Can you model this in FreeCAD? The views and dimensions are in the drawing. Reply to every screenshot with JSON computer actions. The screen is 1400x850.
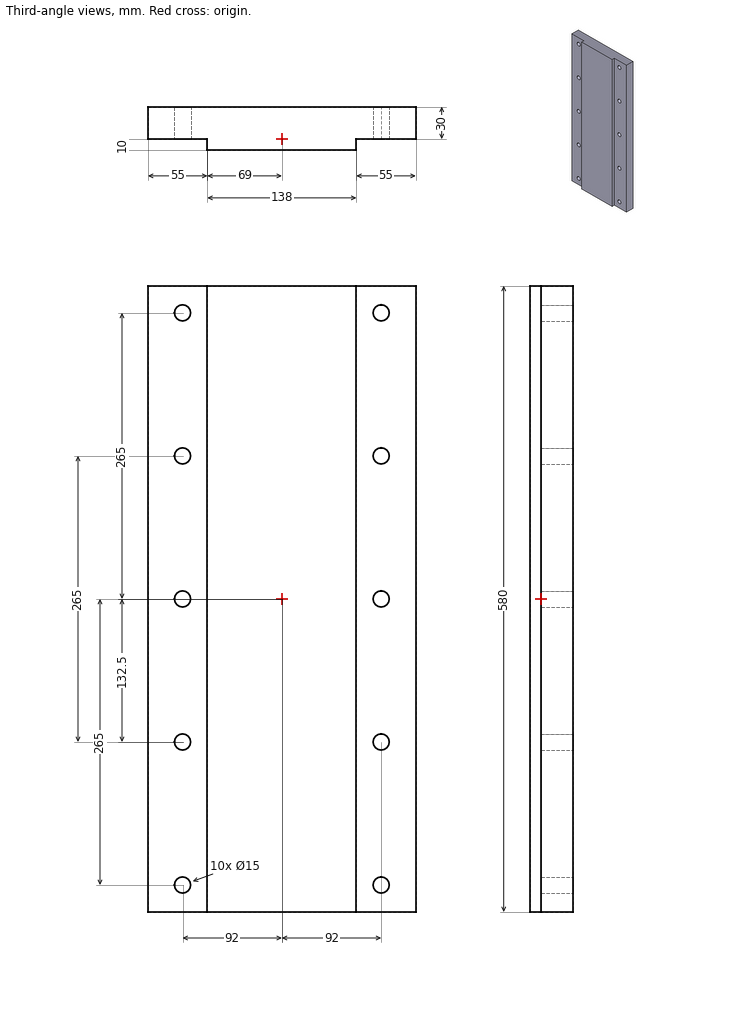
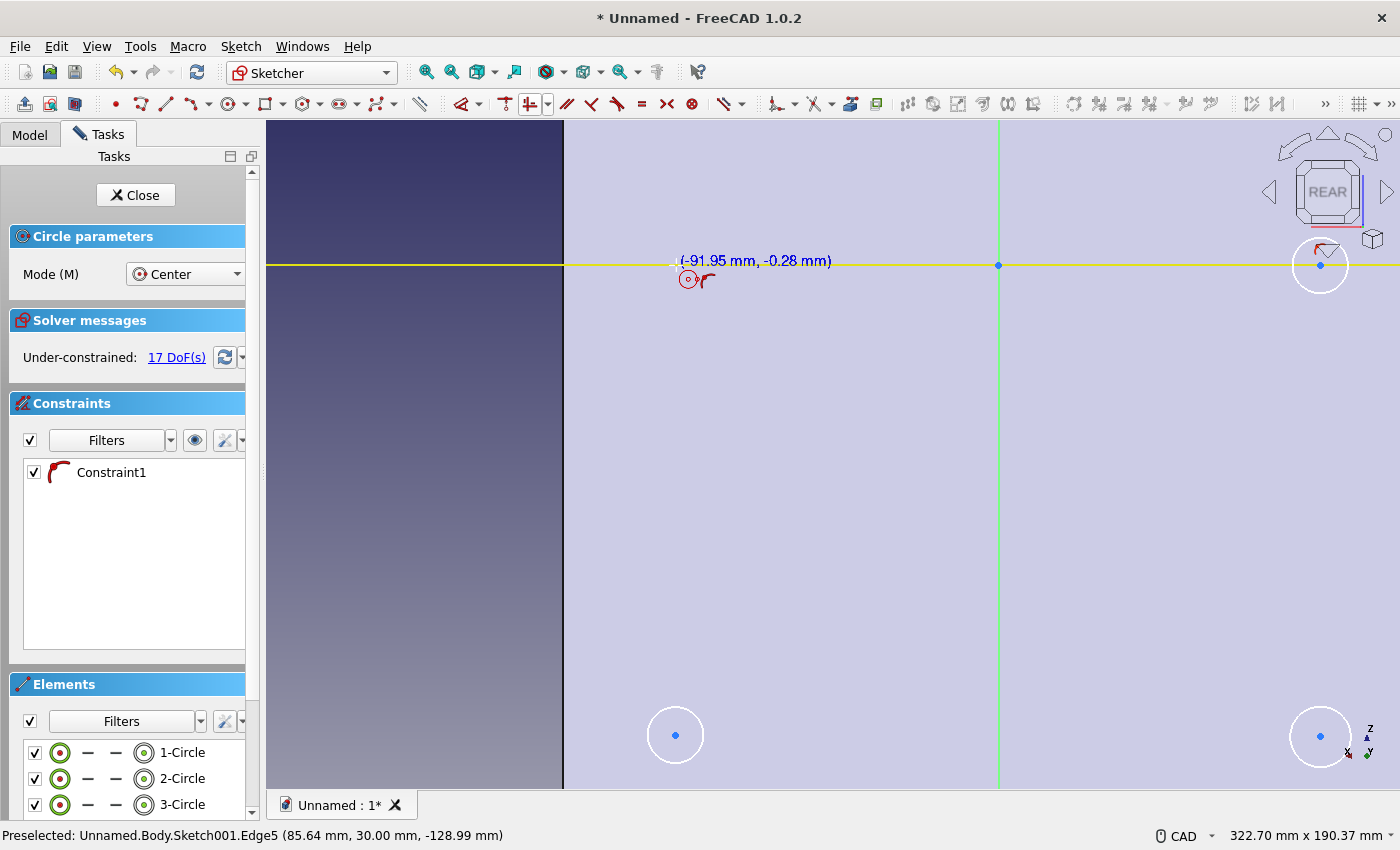
{"action": "scroll", "coordinate": [688, 516], "scroll_direction": "down", "scroll_amount": 7}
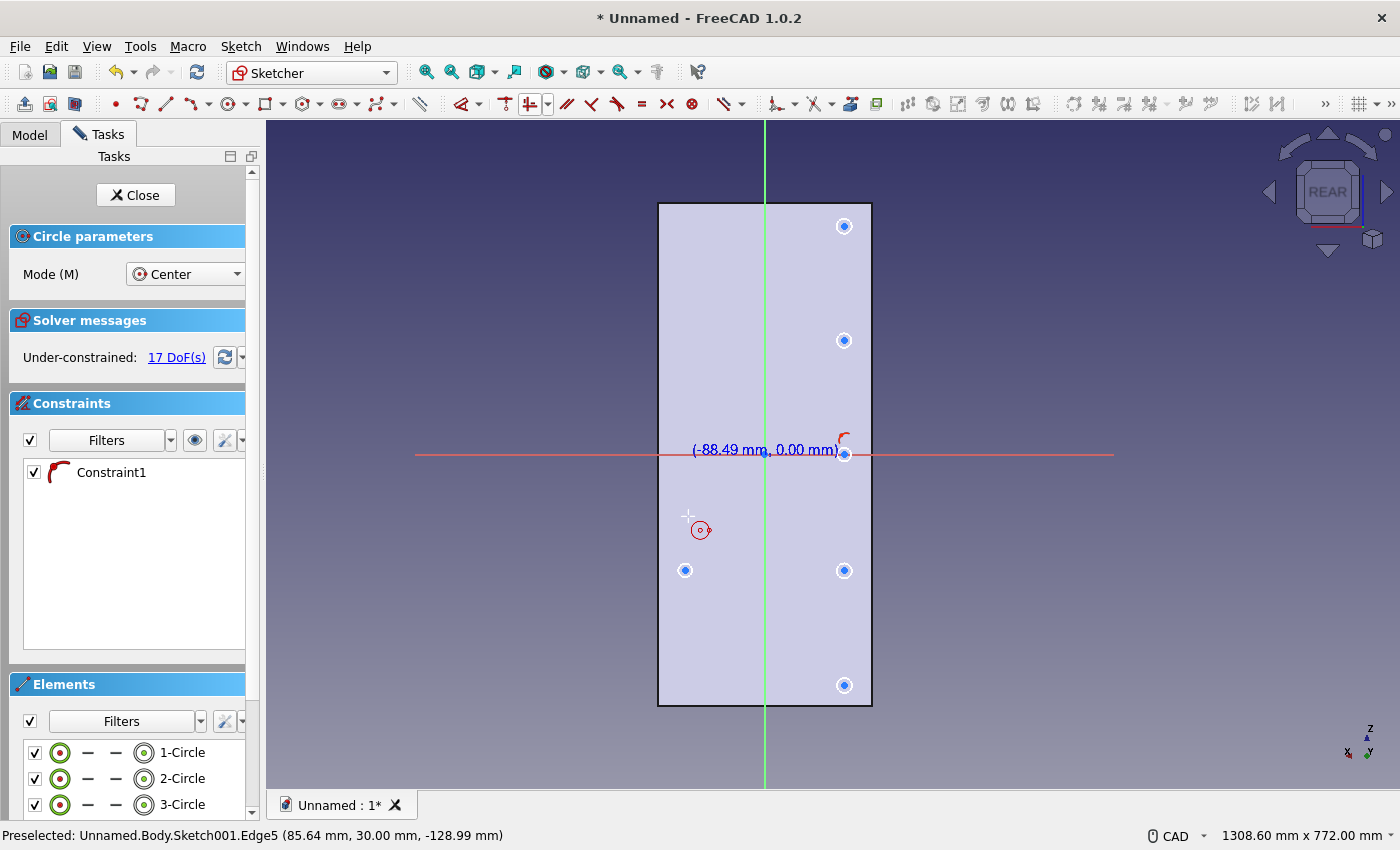
{"action": "left_click", "coordinate": [685, 455]}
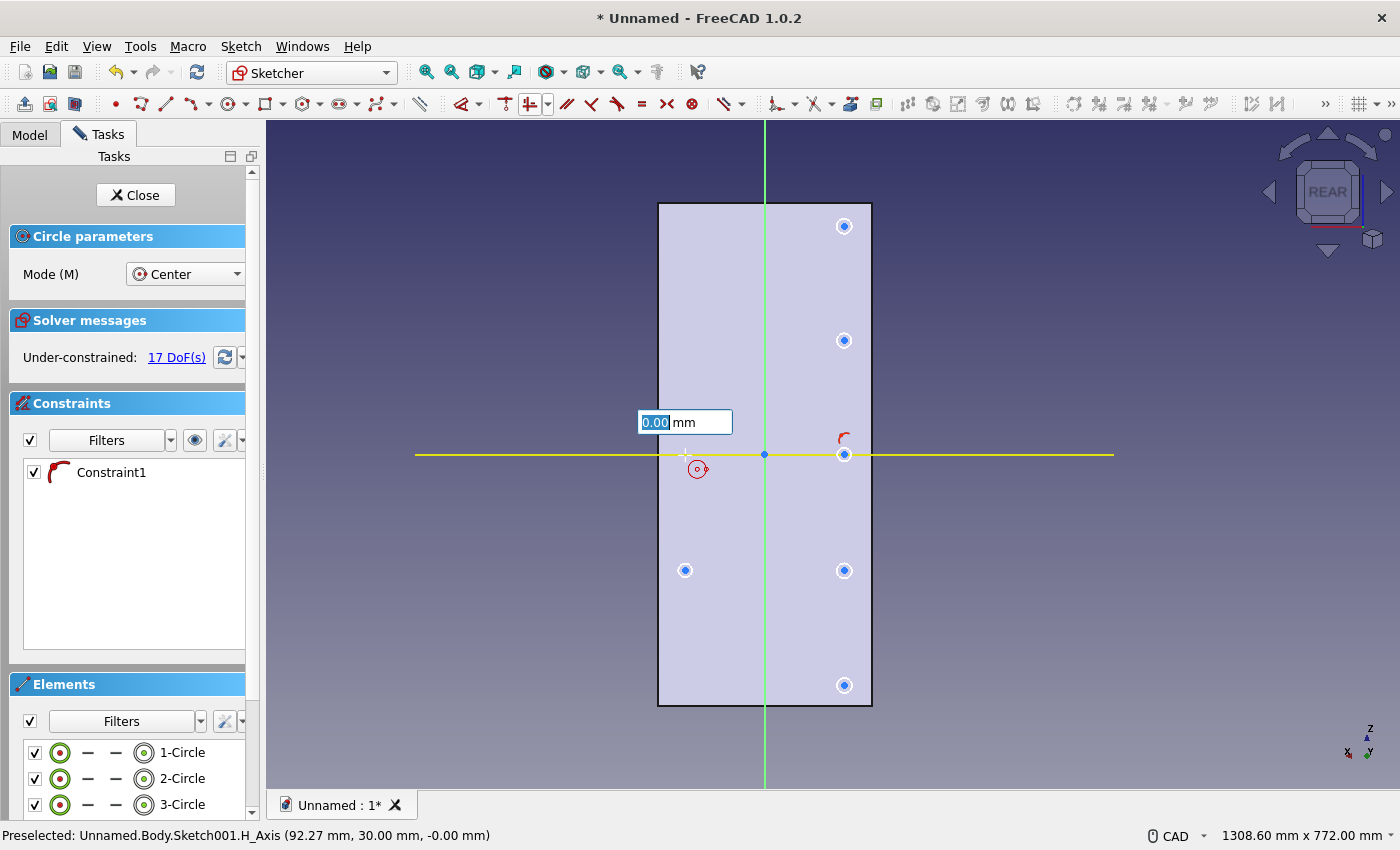
{"action": "scroll", "coordinate": [683, 461], "scroll_direction": "up", "scroll_amount": 5}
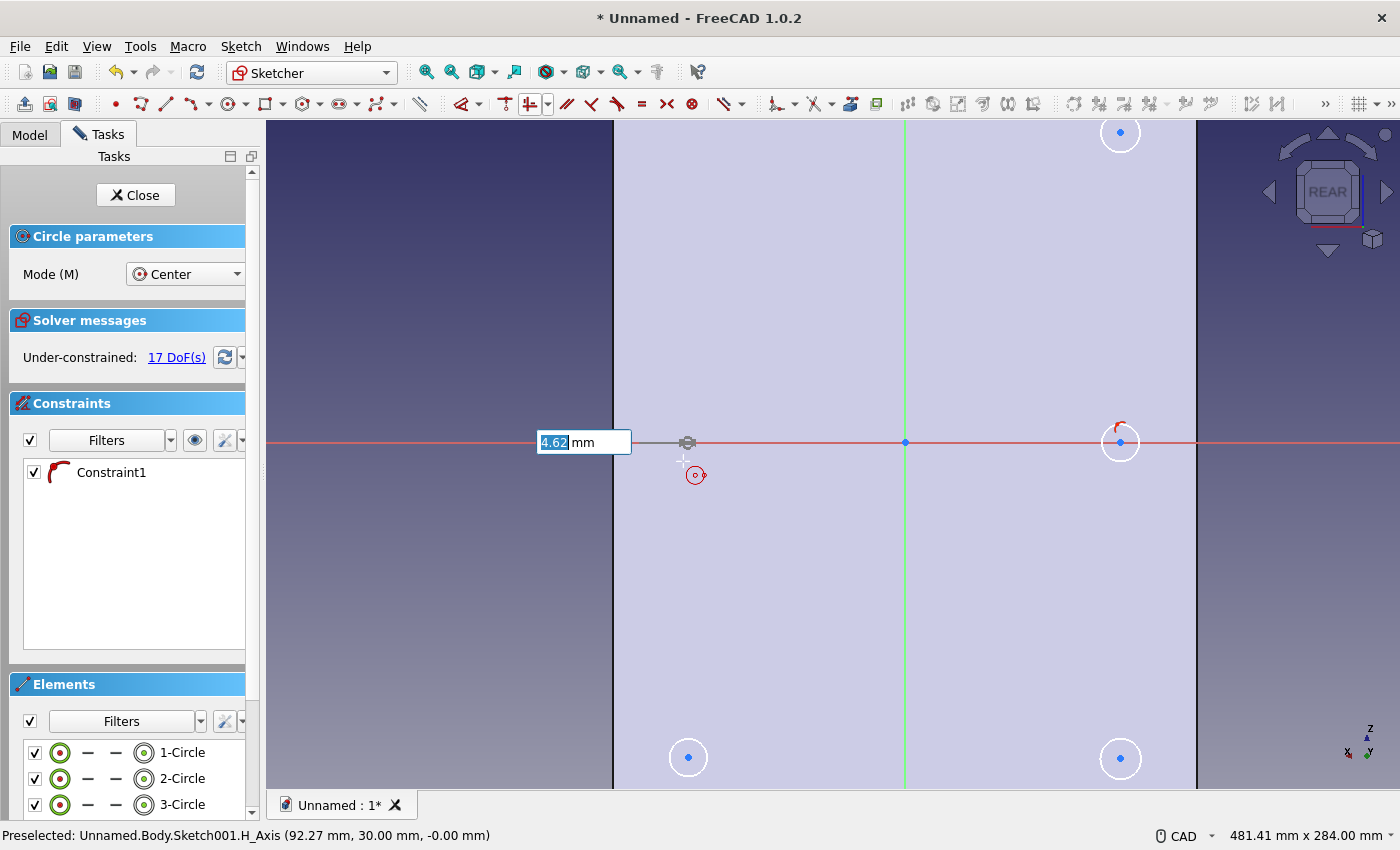
{"action": "left_click", "coordinate": [682, 459]}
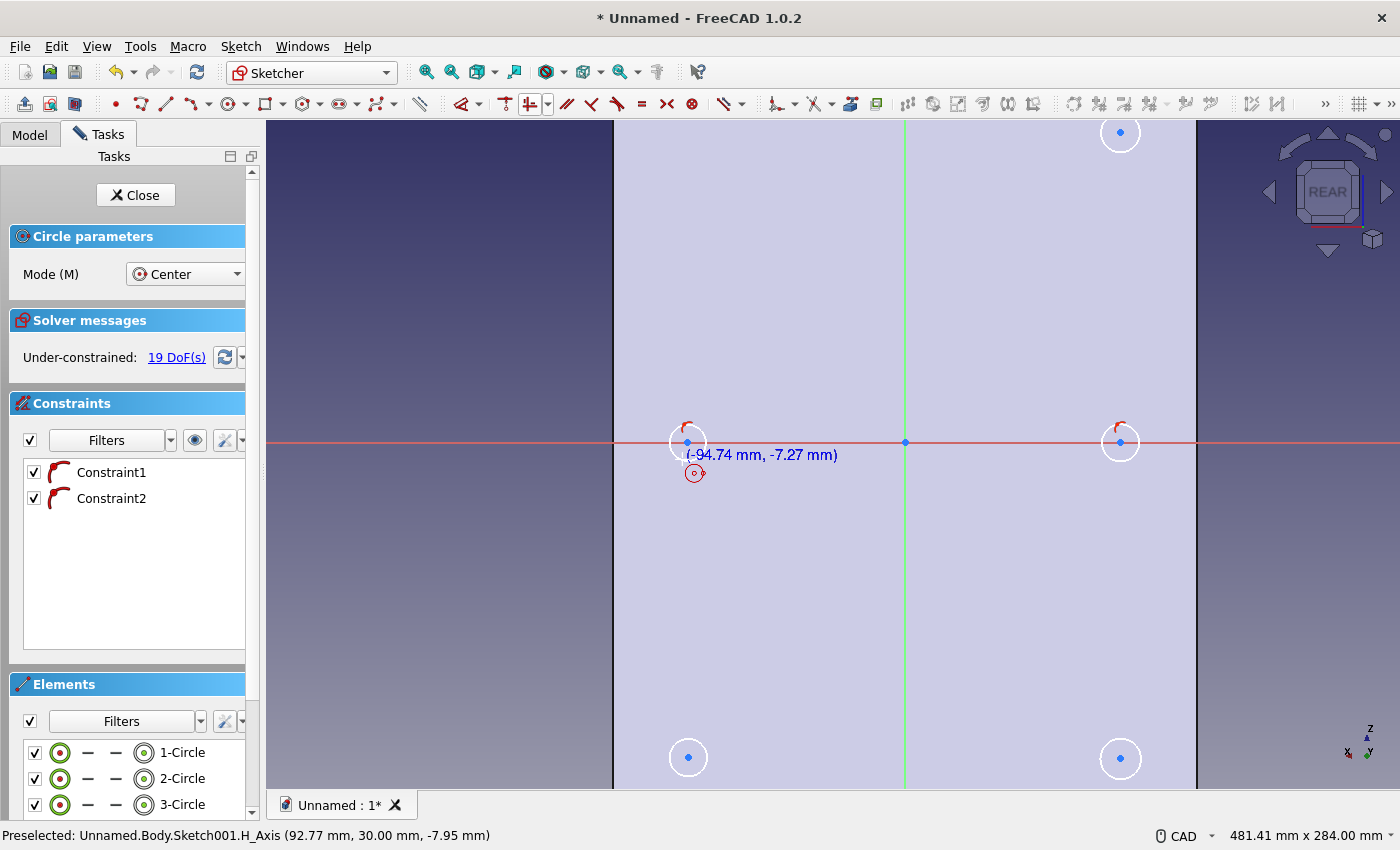
{"action": "scroll", "coordinate": [683, 461], "scroll_direction": "down", "scroll_amount": 5}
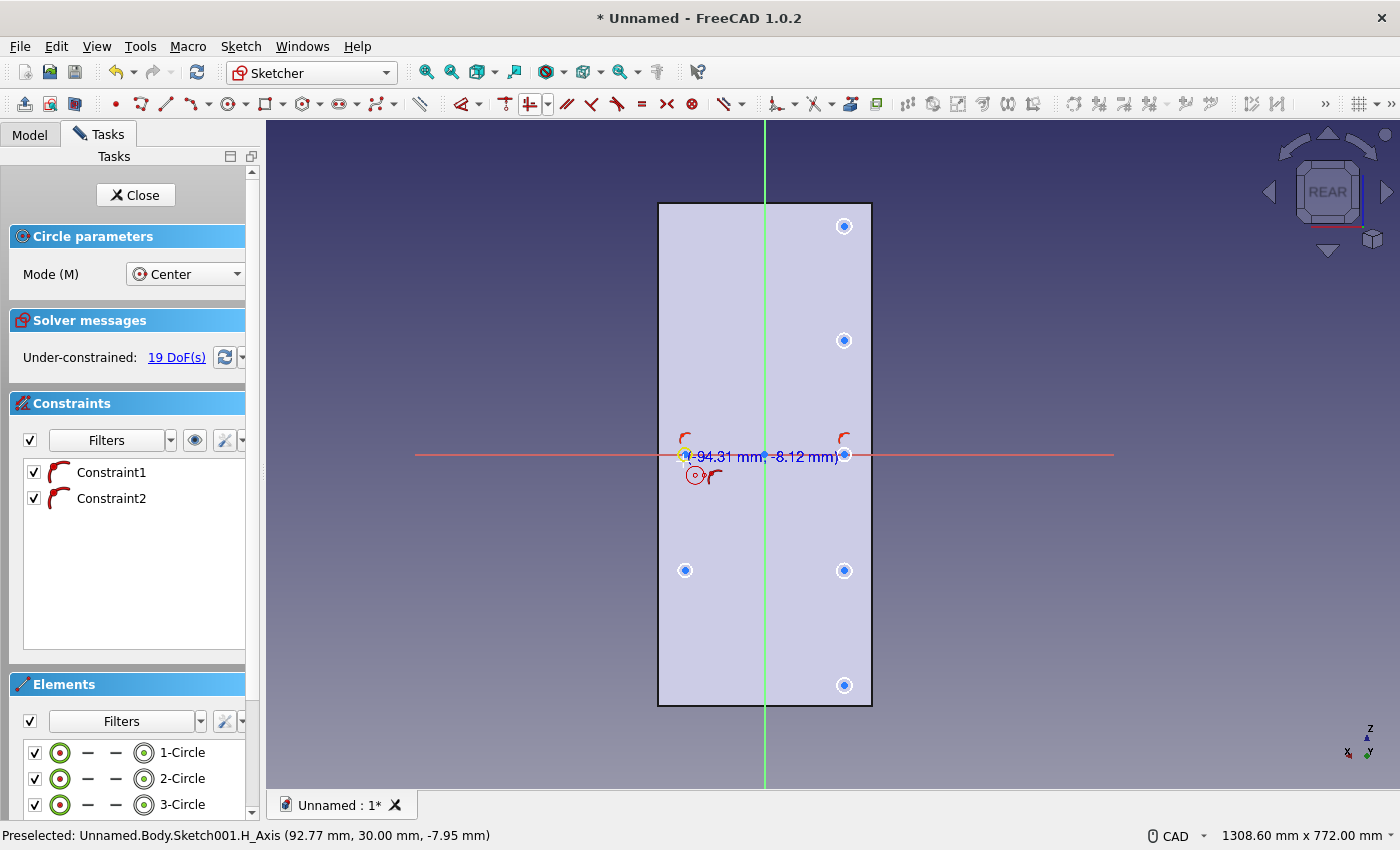
{"action": "scroll", "coordinate": [685, 340], "scroll_direction": "up", "scroll_amount": 7}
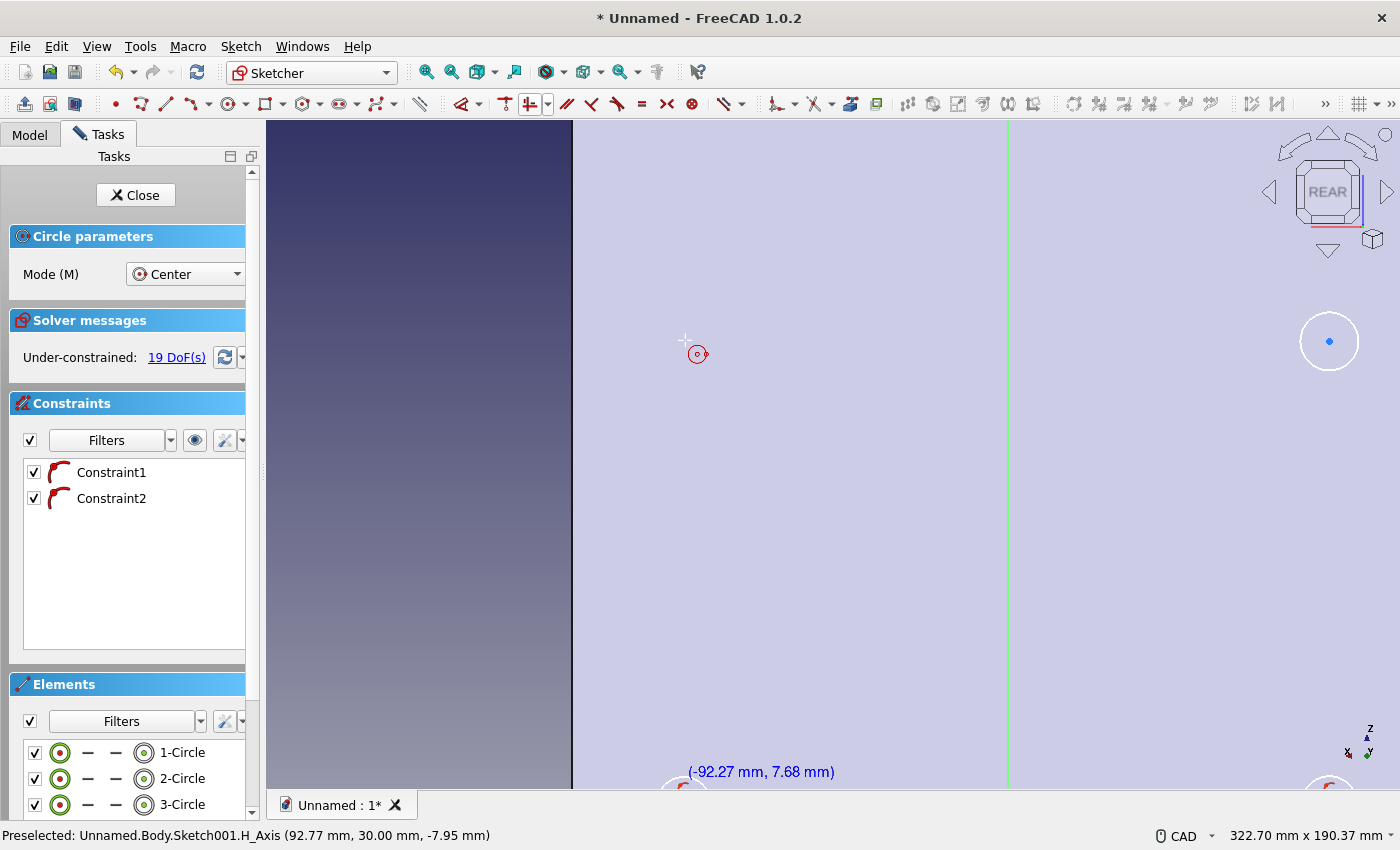
{"action": "scroll", "coordinate": [685, 340], "scroll_direction": "down", "scroll_amount": 7}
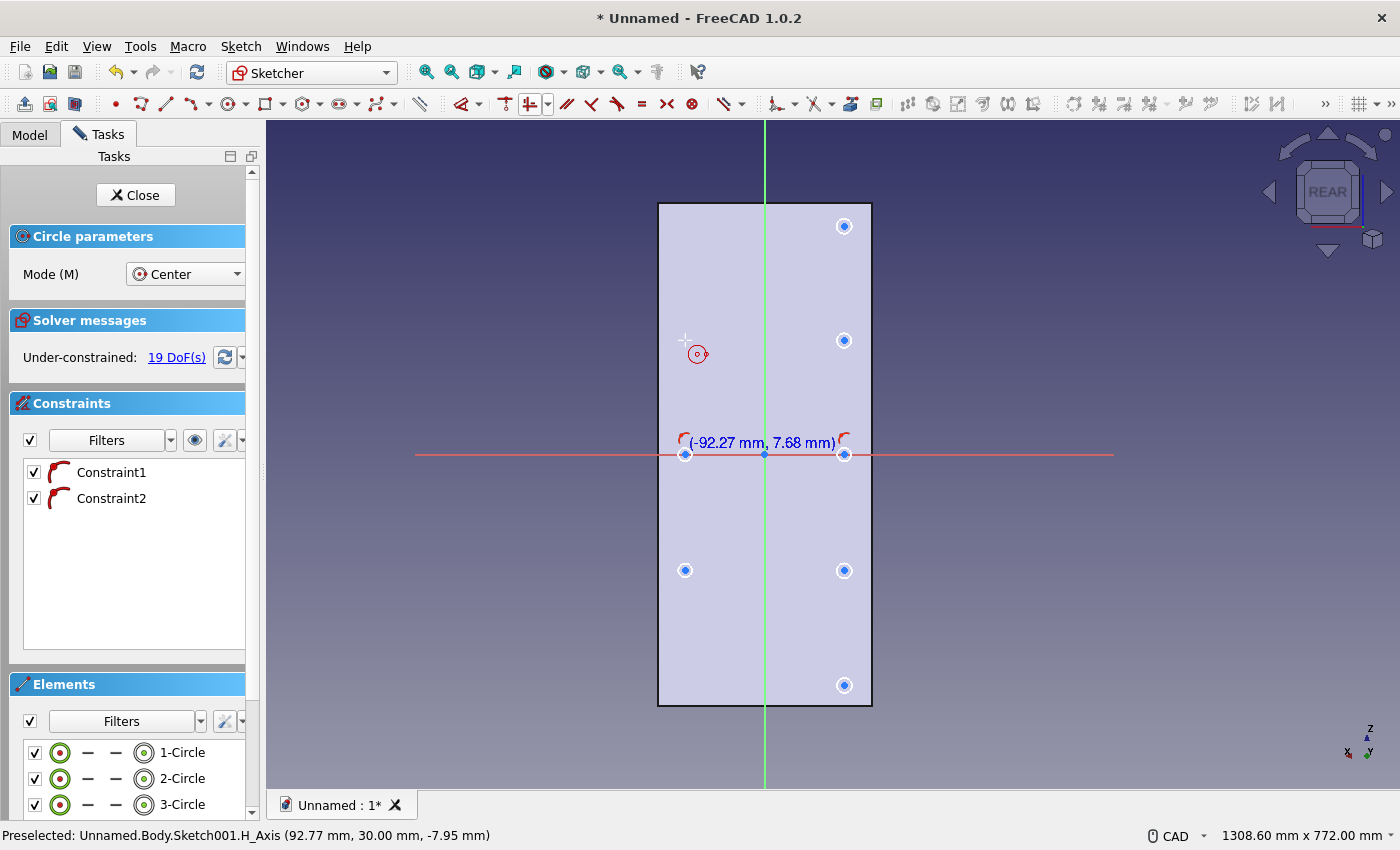
{"action": "left_click", "coordinate": [685, 340]}